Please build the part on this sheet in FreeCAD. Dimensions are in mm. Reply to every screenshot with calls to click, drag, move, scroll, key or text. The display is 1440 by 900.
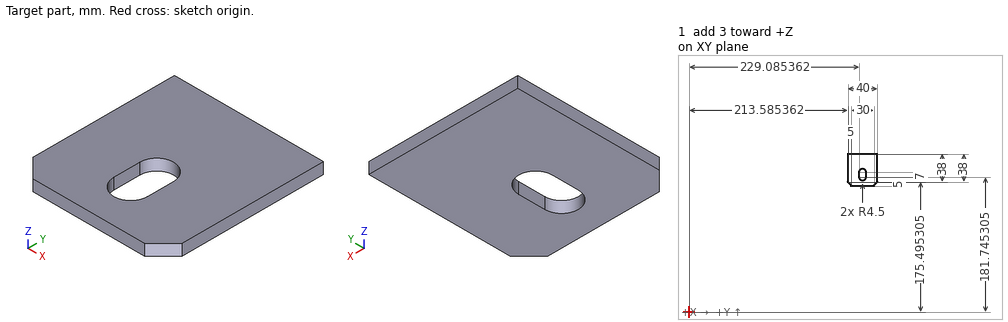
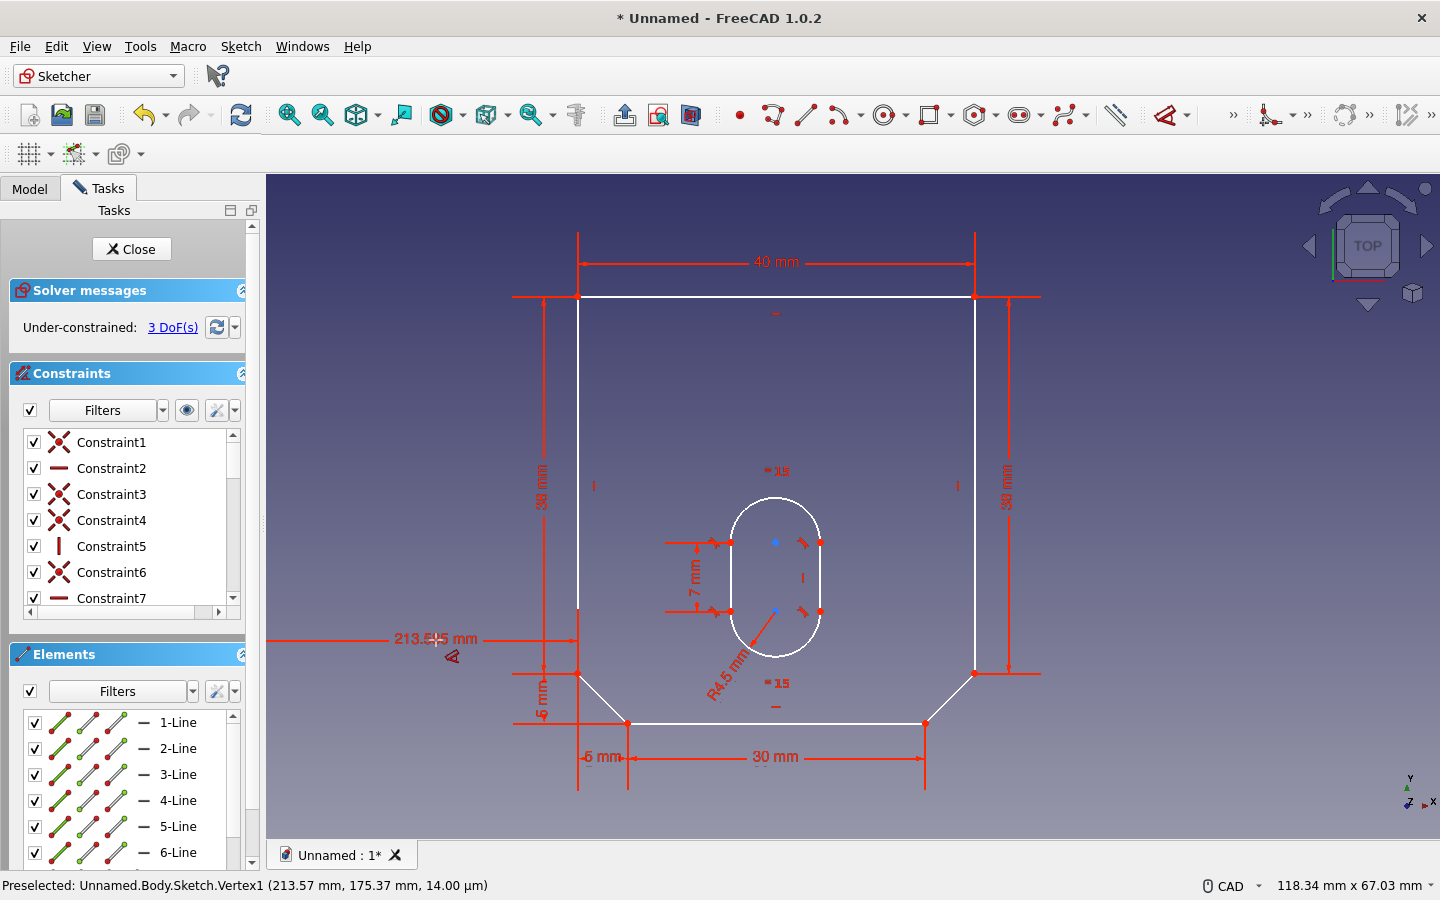
click(578, 674)
click(612, 790)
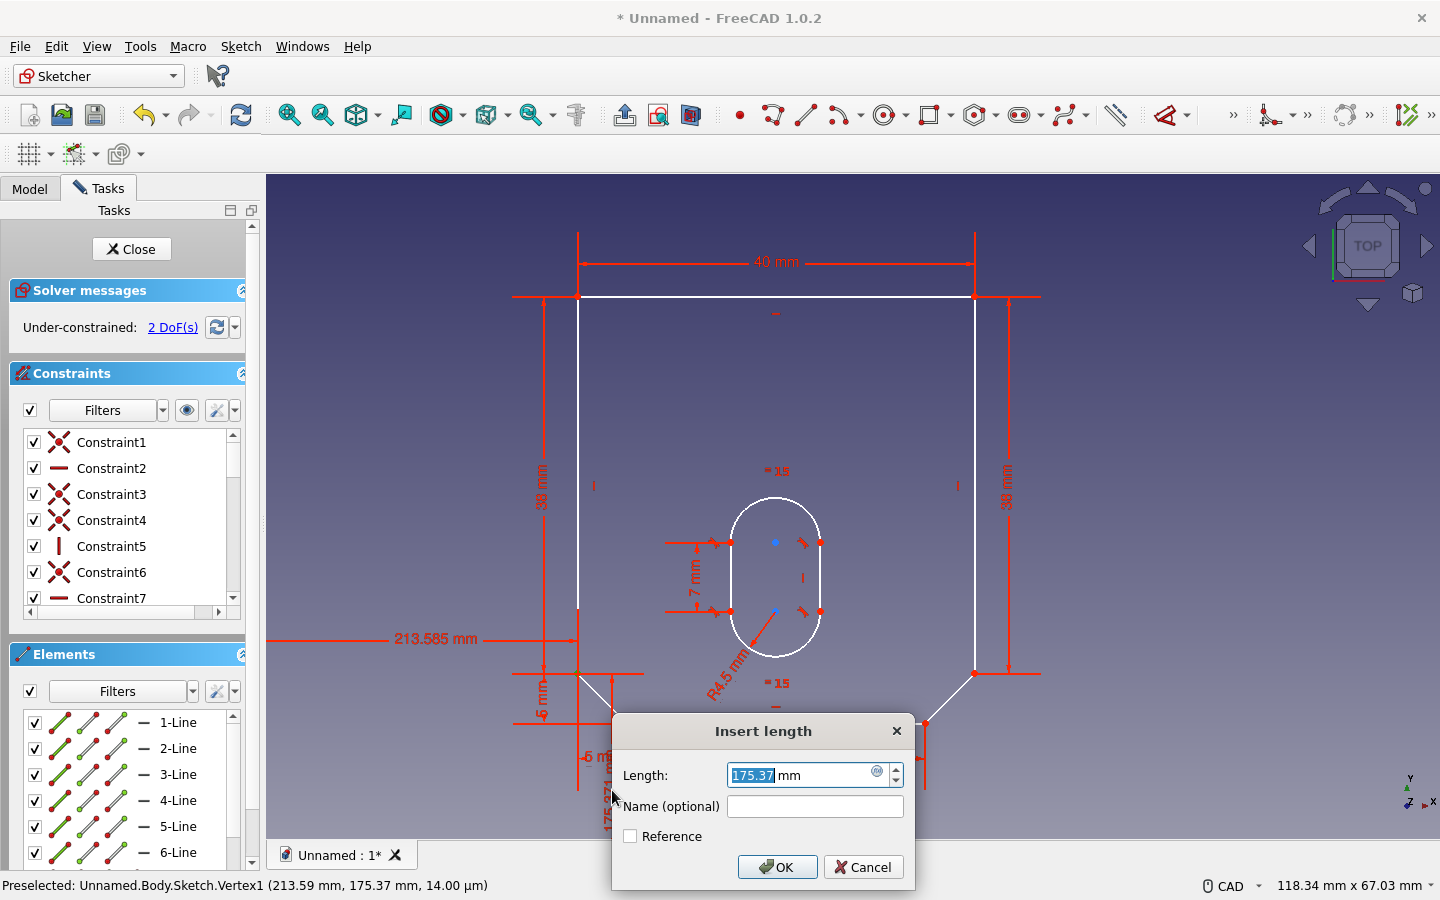
text(175.495305)
key(Return)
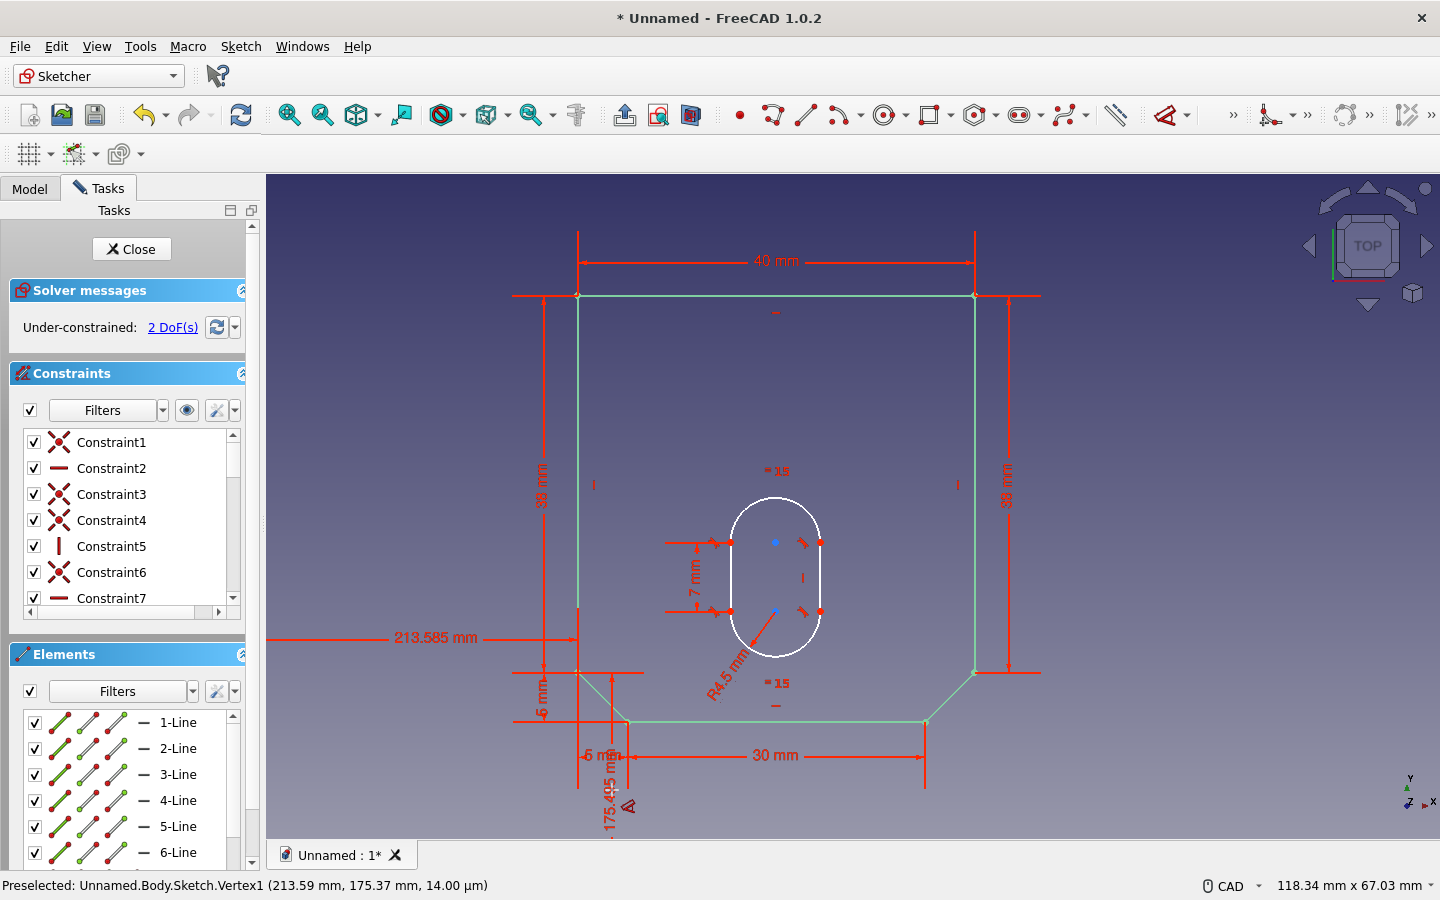
click(731, 612)
click(512, 578)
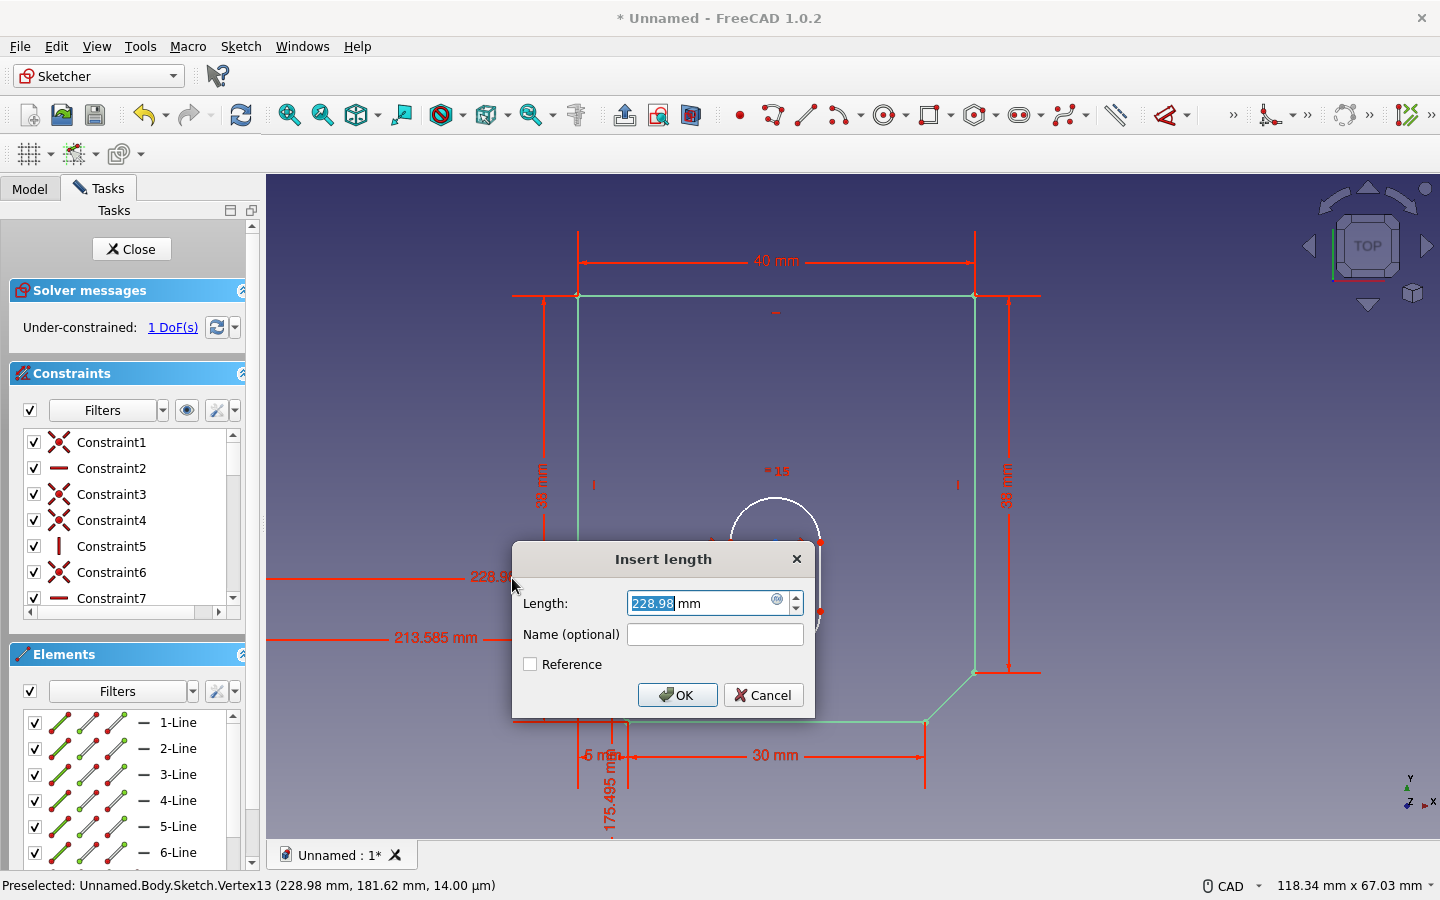
text(229.085362)
key(Return)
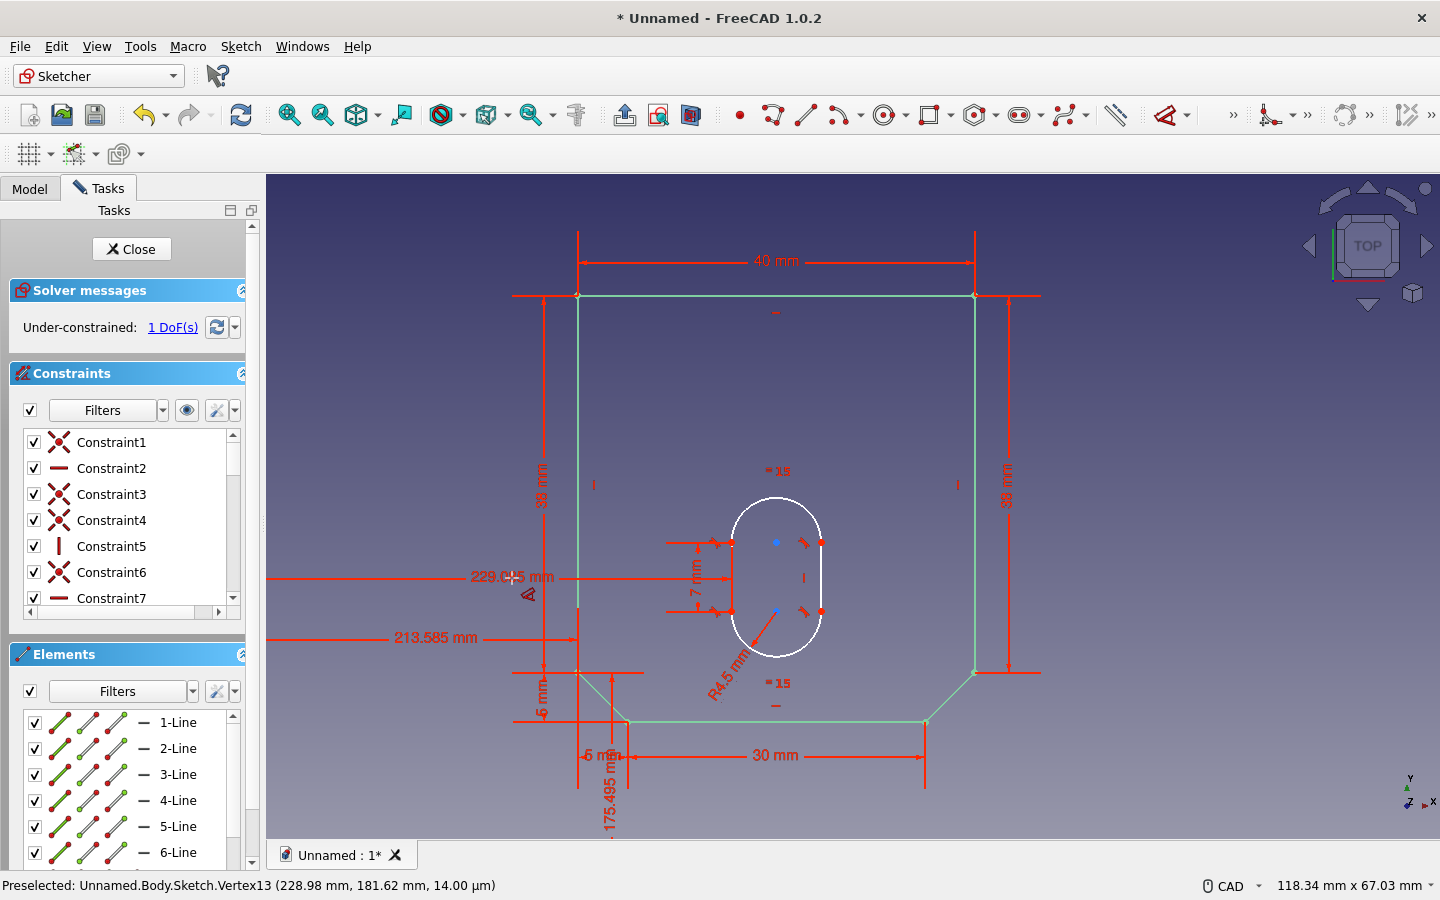
click(732, 612)
click(766, 781)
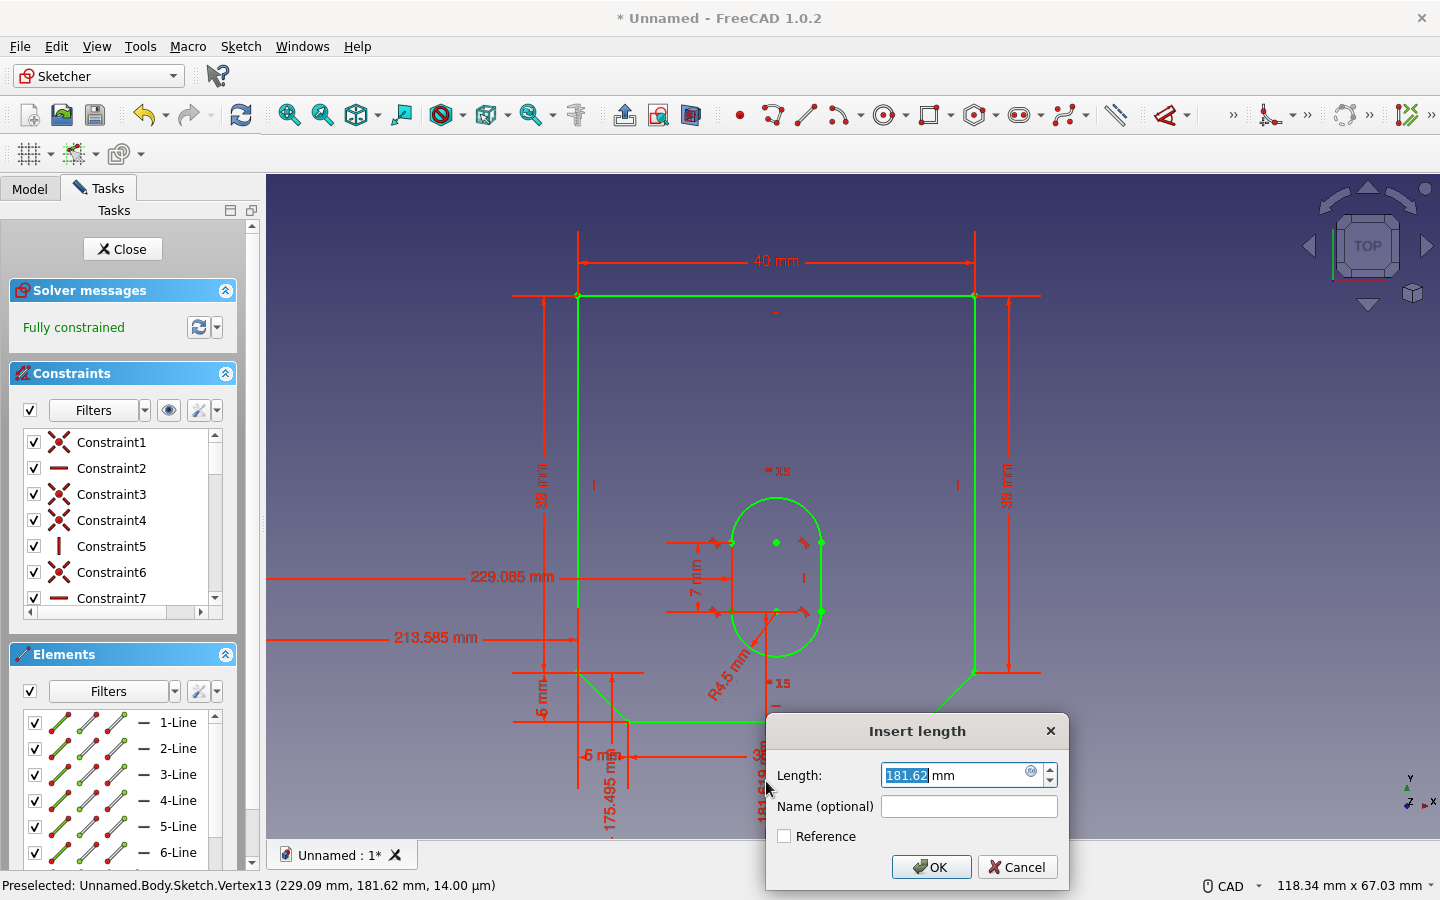
text(181.745305)
key(Return)
key(Escape)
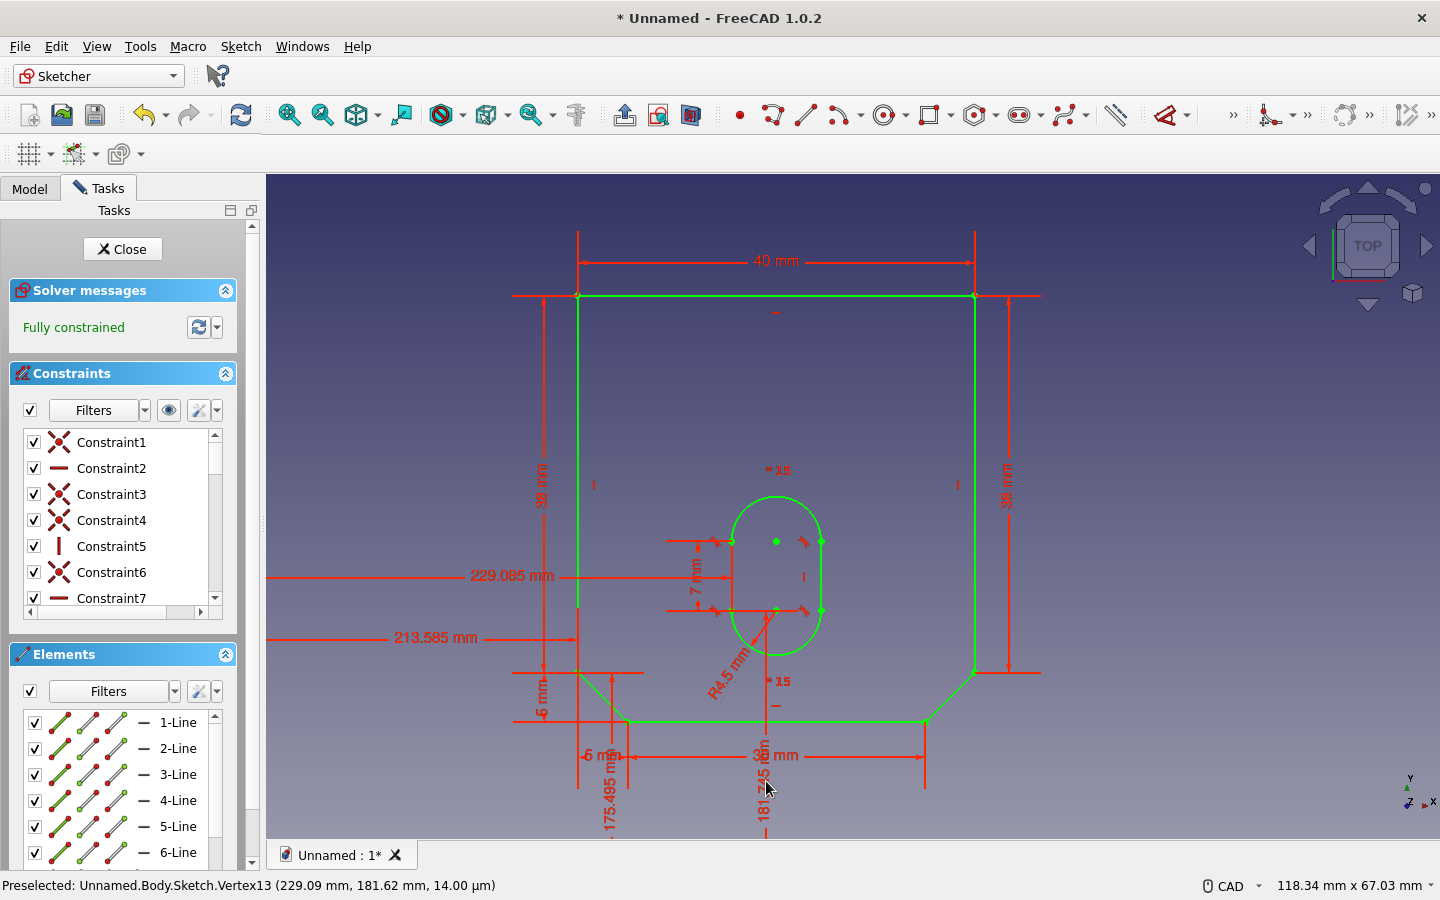
click(123, 249)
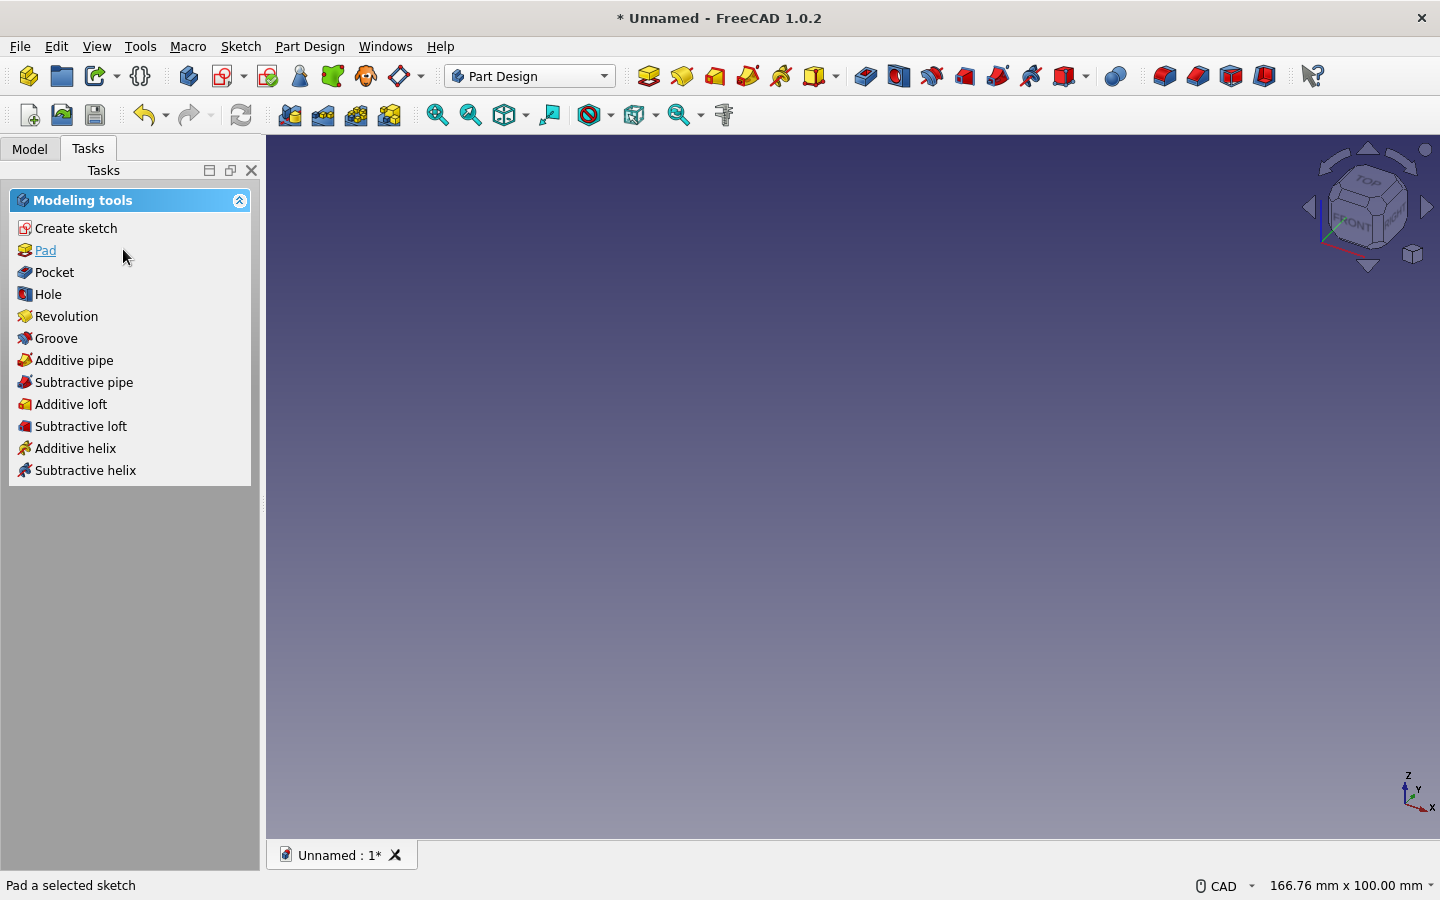
click(649, 76)